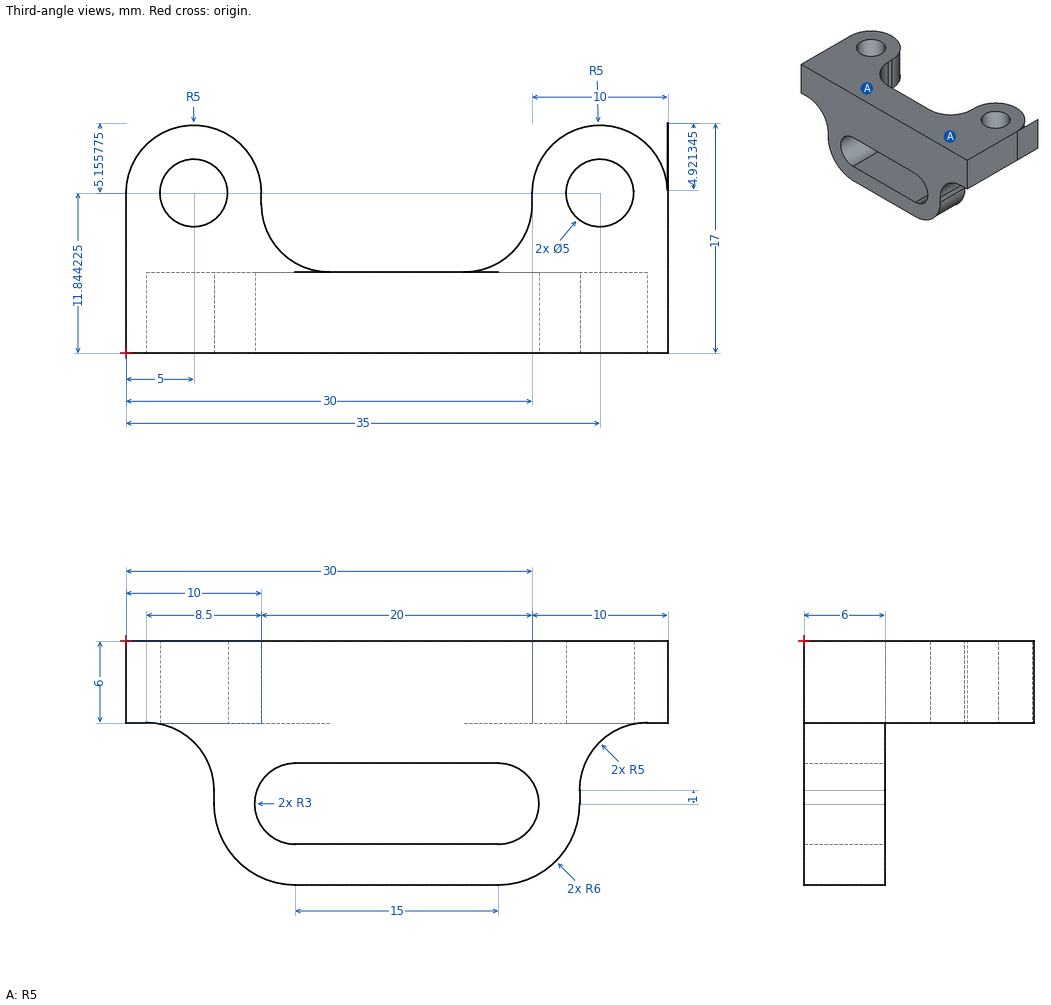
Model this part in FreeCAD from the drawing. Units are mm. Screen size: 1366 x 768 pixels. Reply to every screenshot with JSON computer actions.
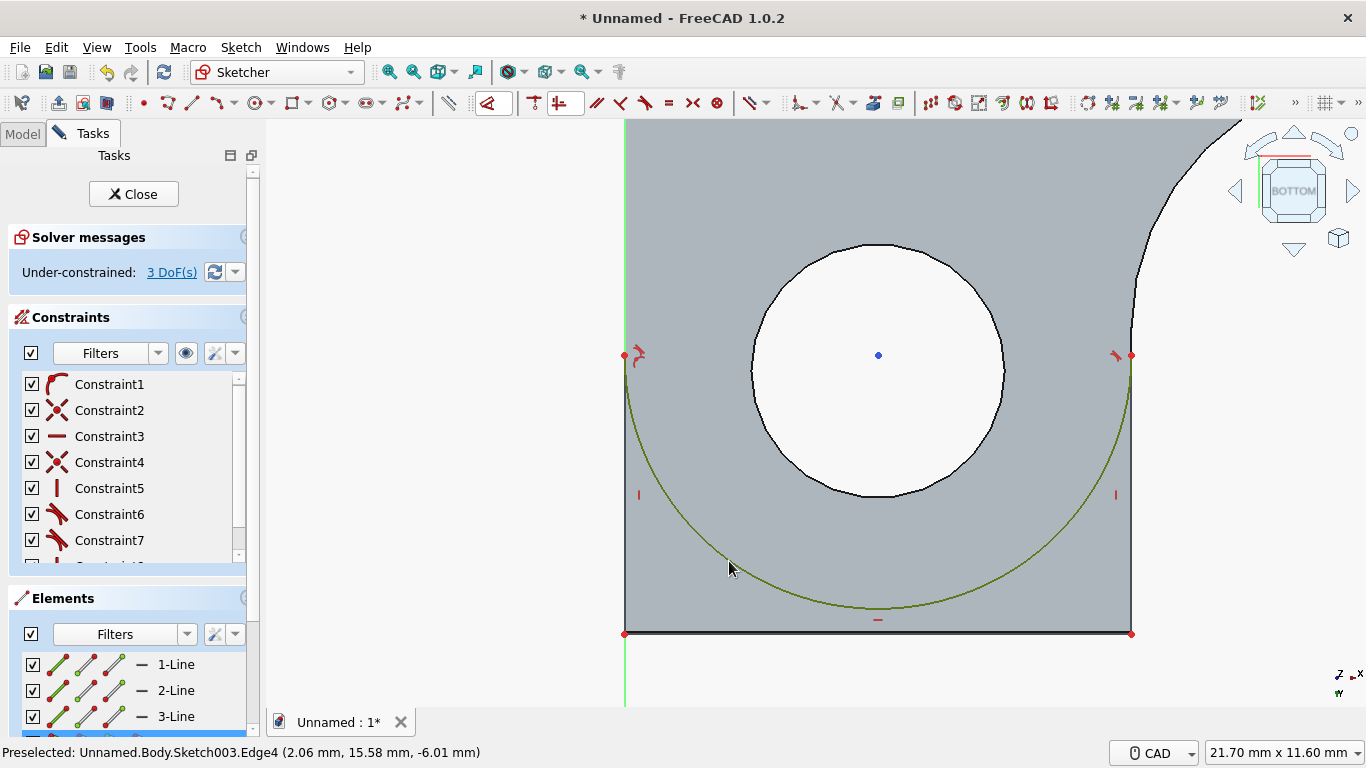
{"action": "key", "text": "k r"}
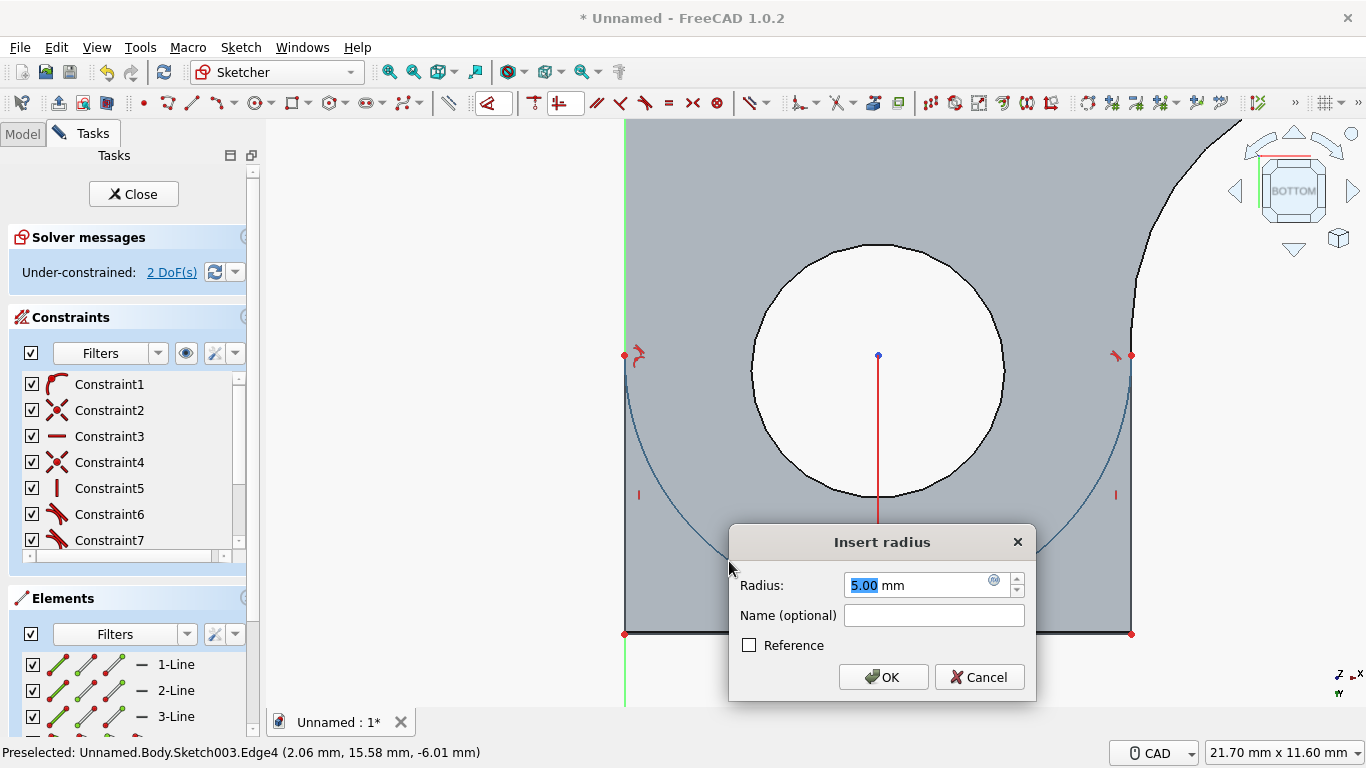
{"action": "type", "text": "5"}
{"action": "key", "text": "Return"}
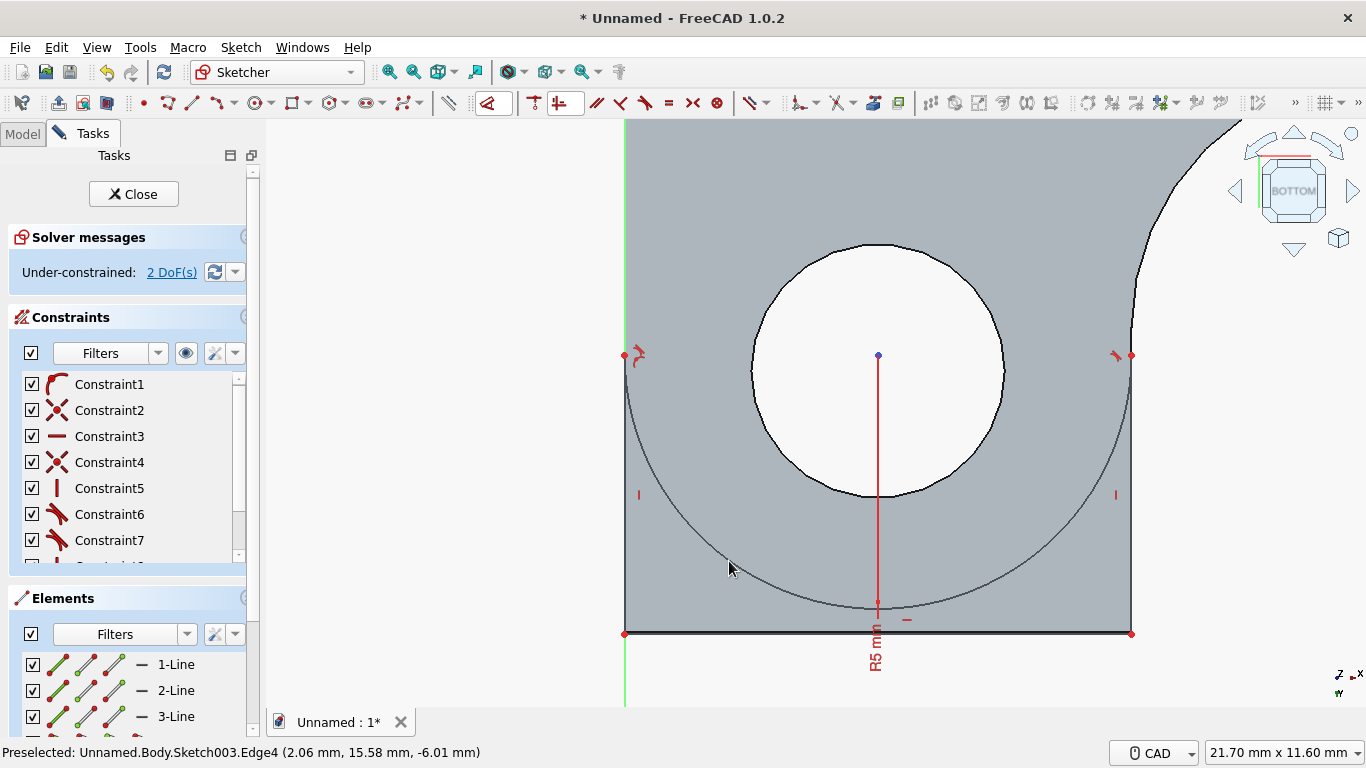
{"action": "left_click", "coordinate": [625, 634]}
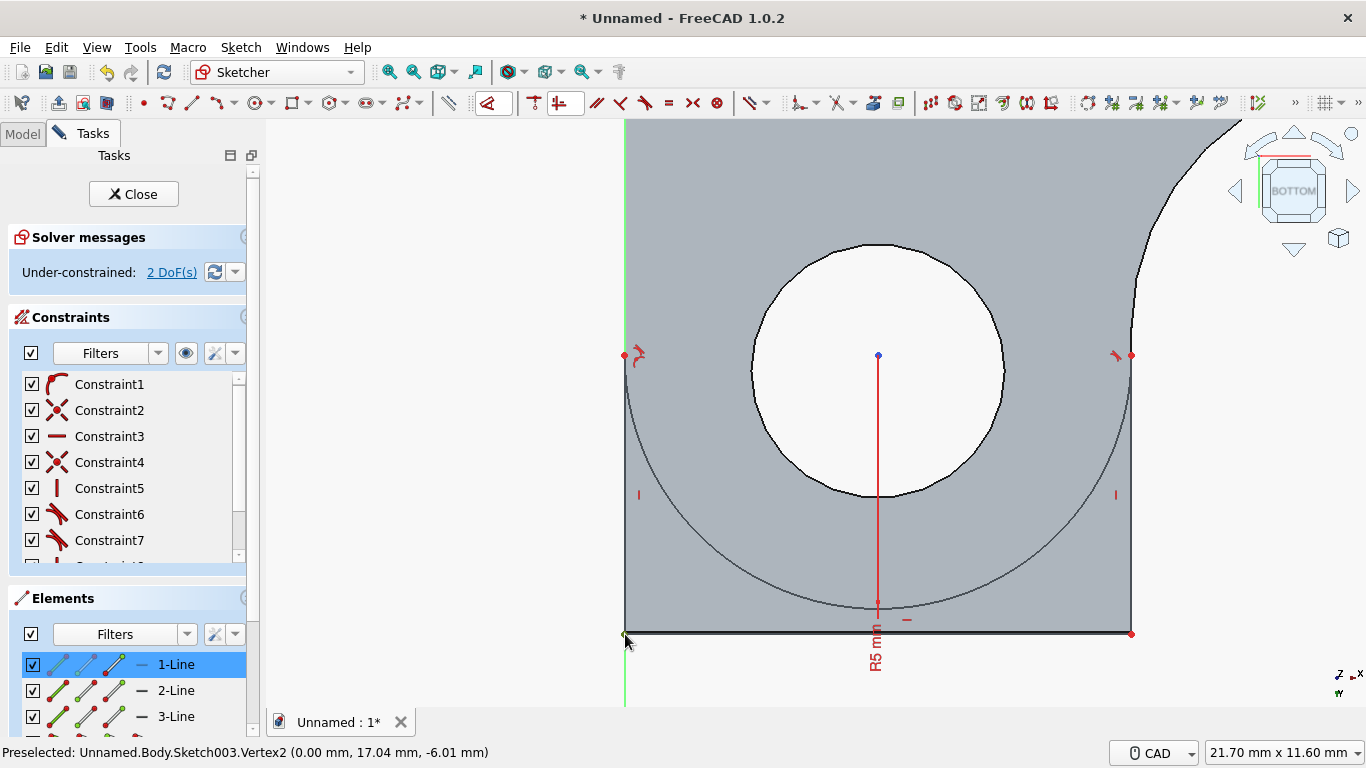
{"action": "key", "text": "i"}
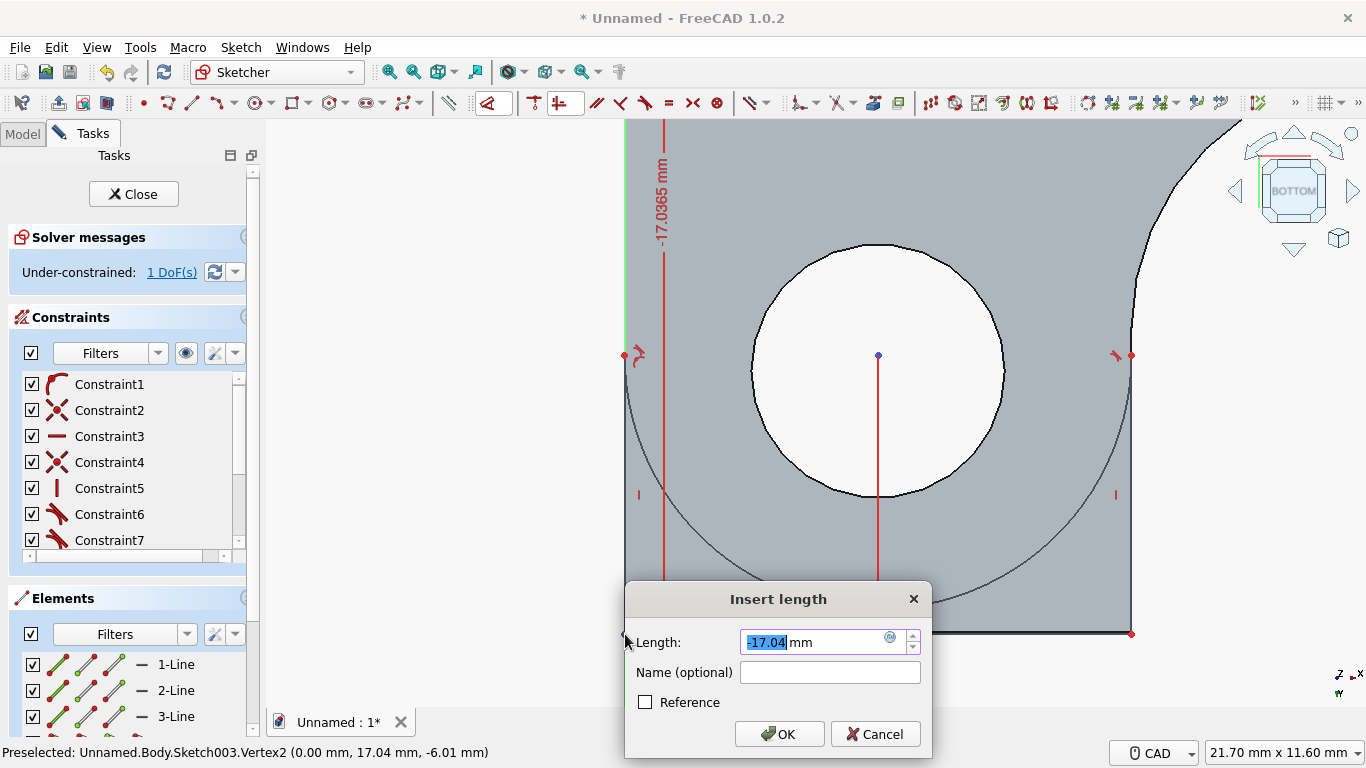
{"action": "type", "text": "-17"}
{"action": "key", "text": "Return"}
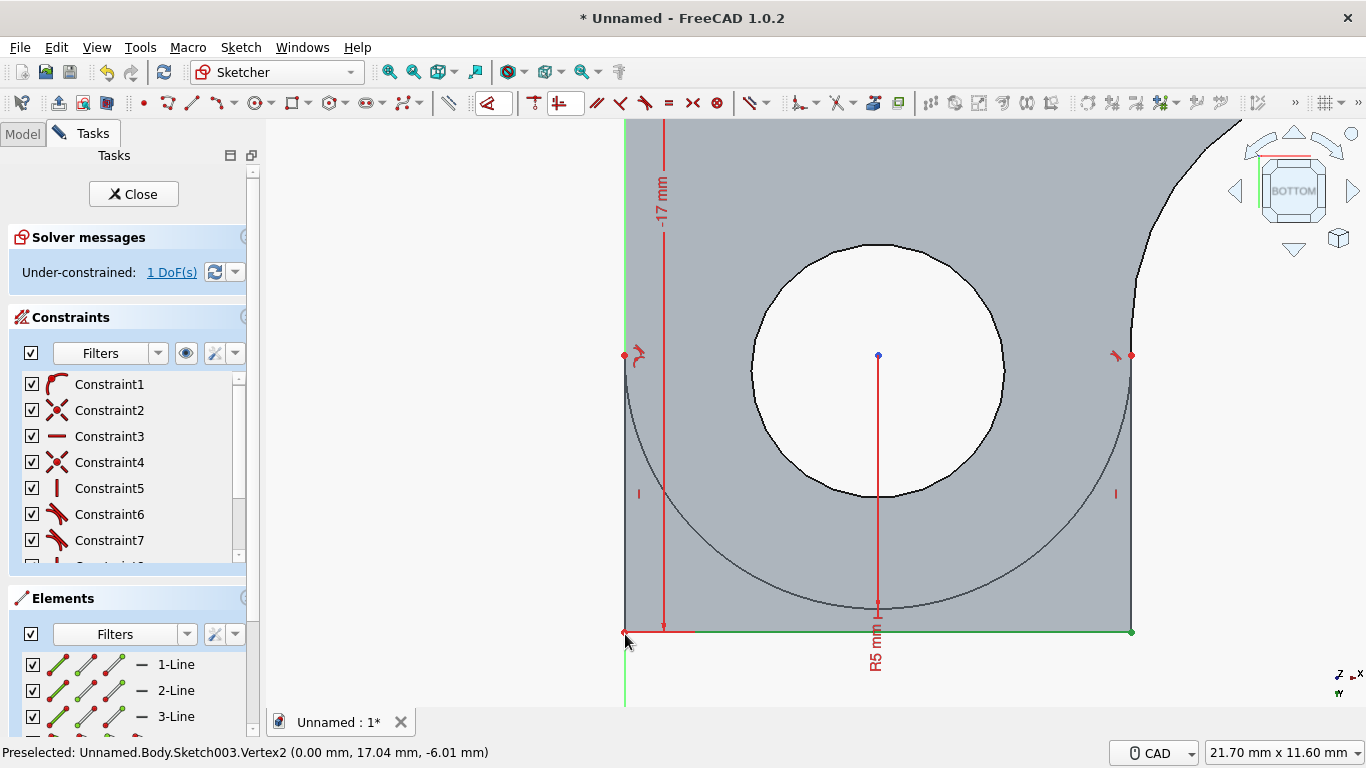
{"action": "left_click", "coordinate": [625, 439]}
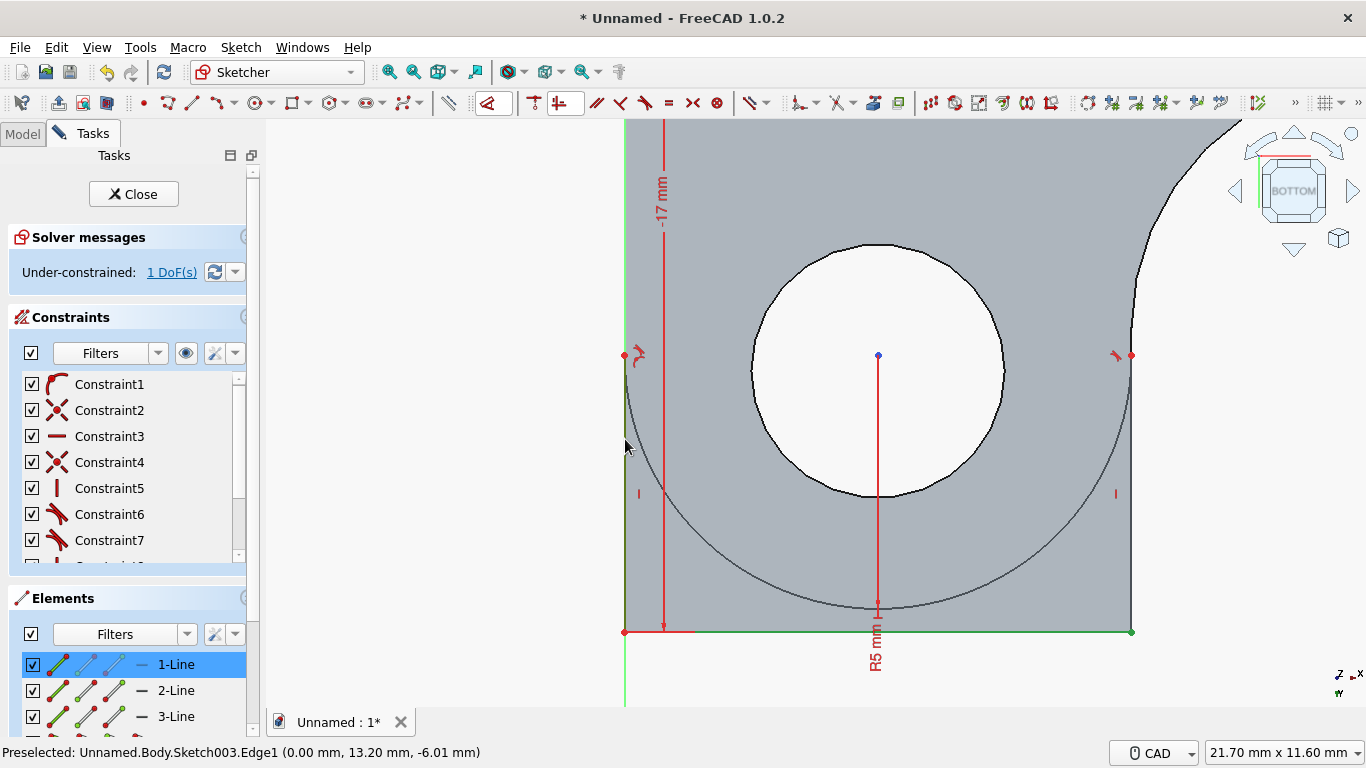
{"action": "key", "text": "i"}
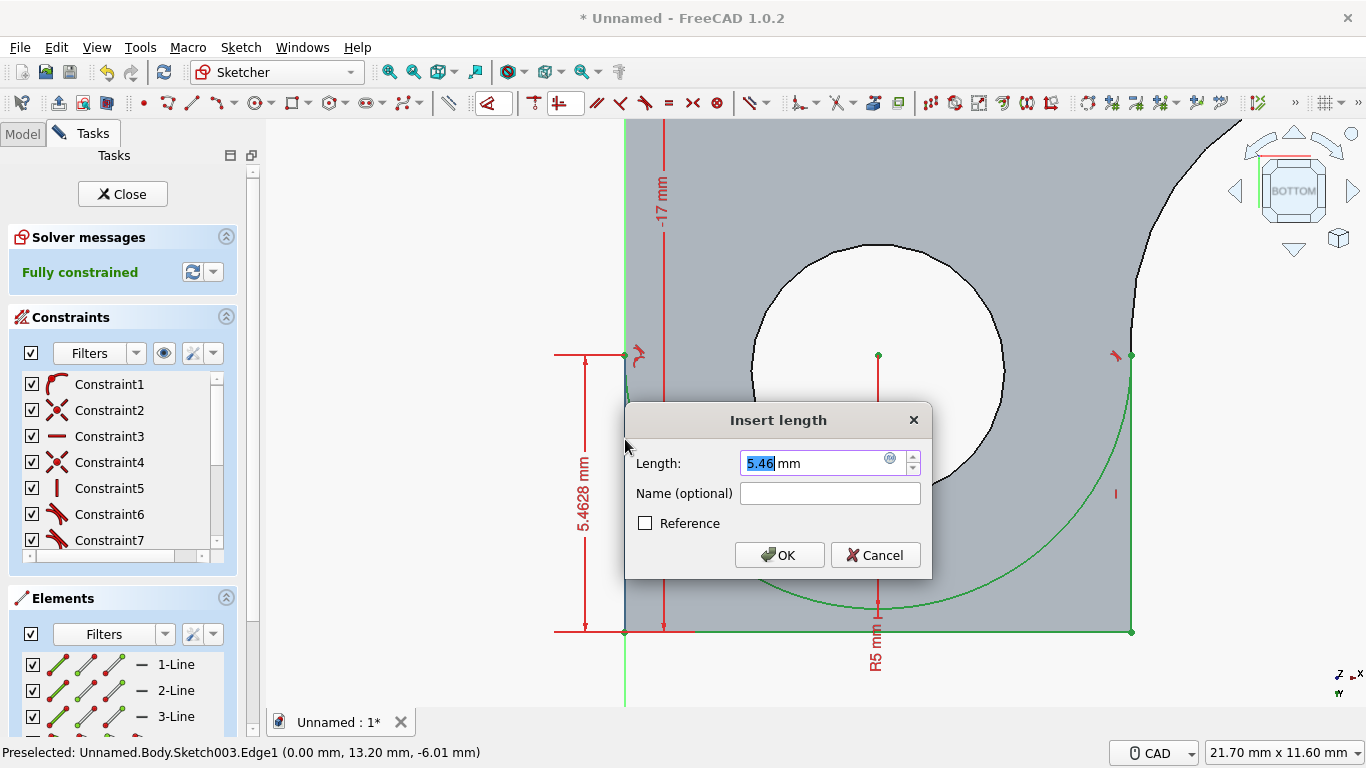
{"action": "type", "text": "5.155775"}
{"action": "key", "text": "Return"}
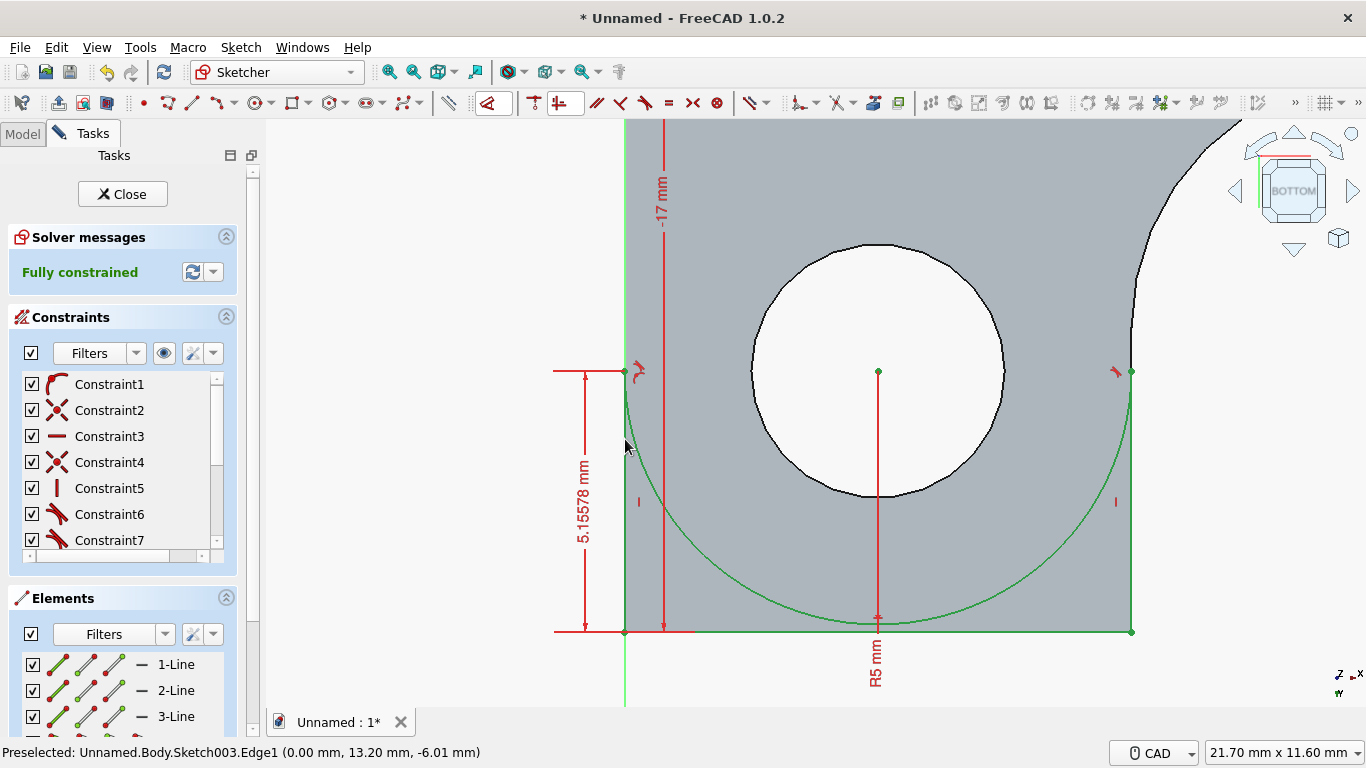
{"action": "left_click", "coordinate": [123, 194]}